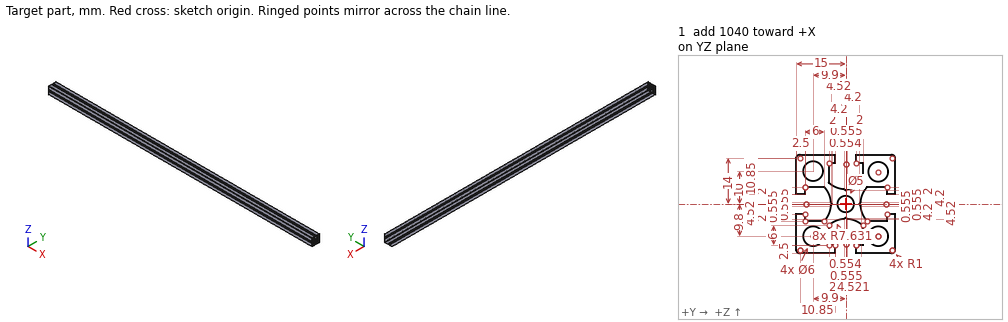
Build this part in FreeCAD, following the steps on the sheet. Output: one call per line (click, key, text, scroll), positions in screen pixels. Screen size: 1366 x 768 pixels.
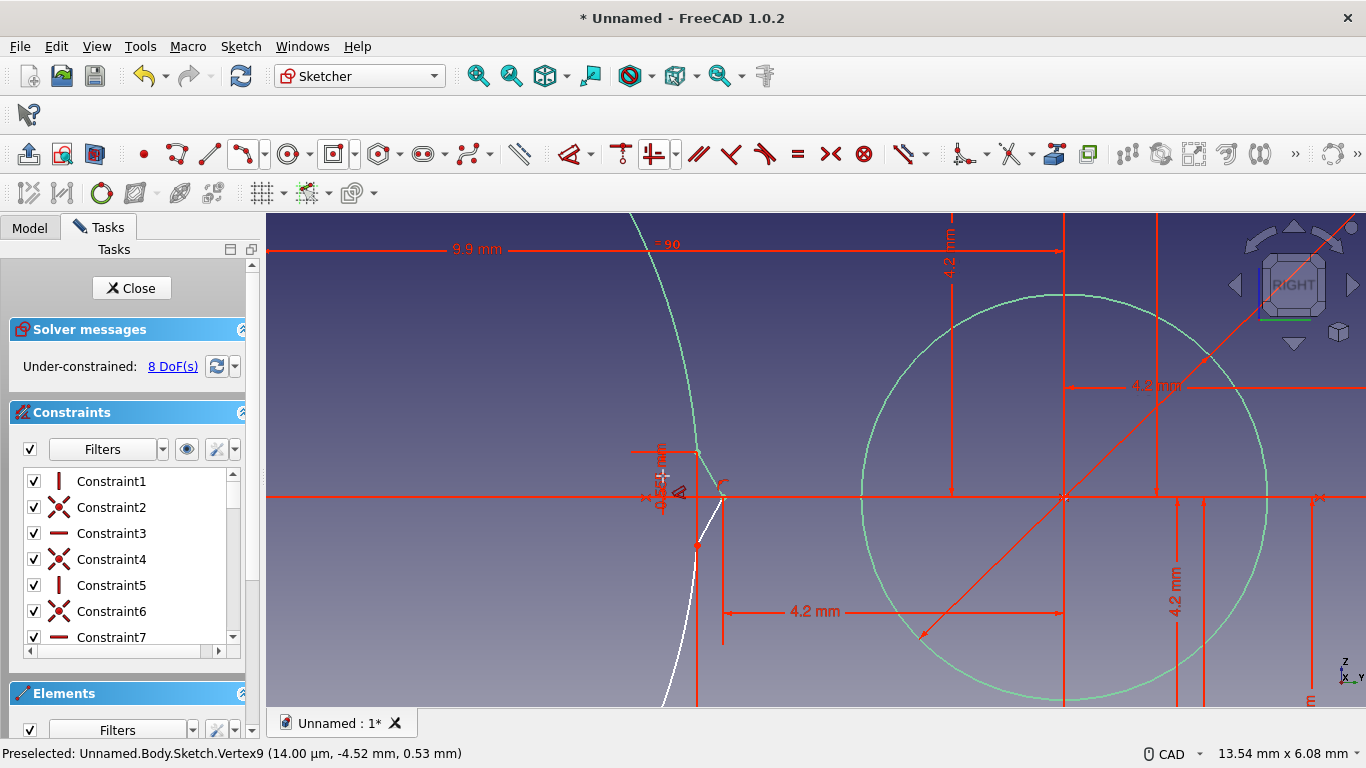
click(697, 545)
click(663, 521)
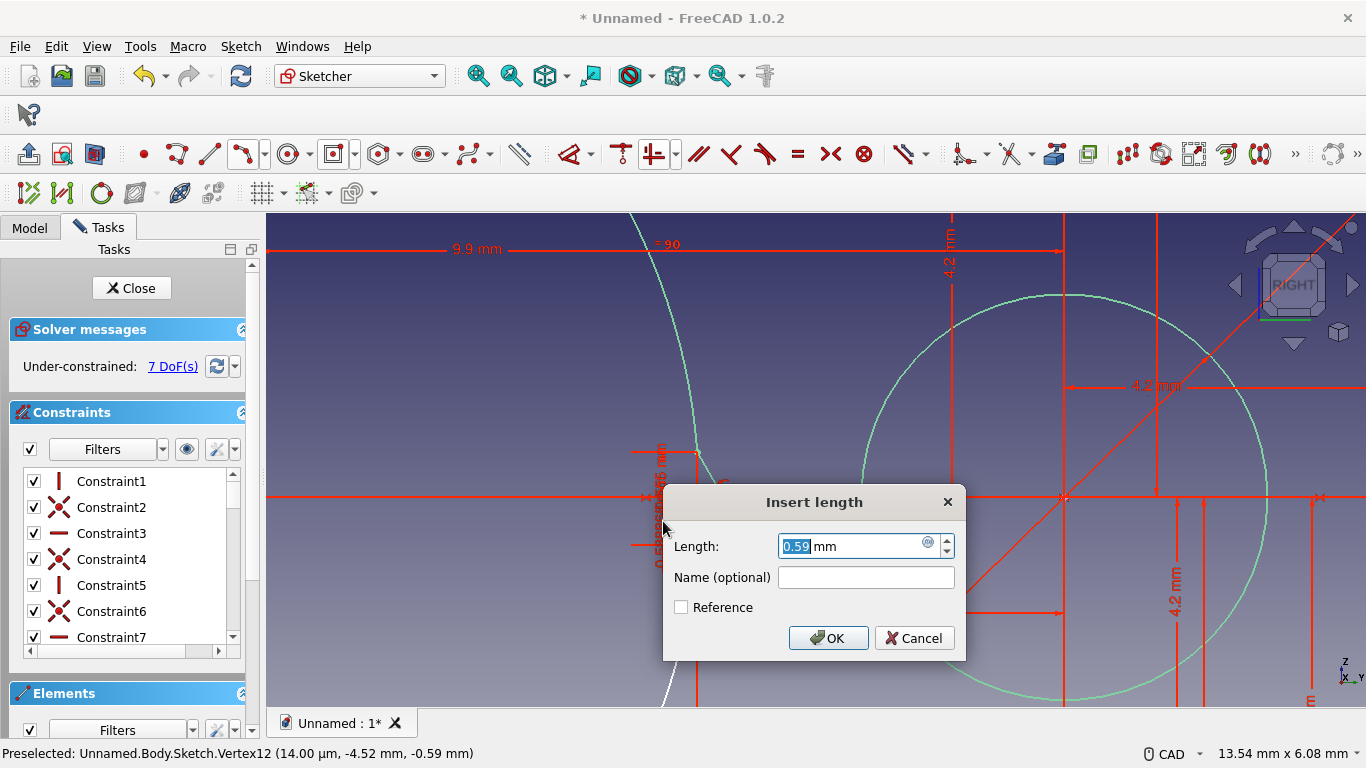
text(0.555)
key(Return)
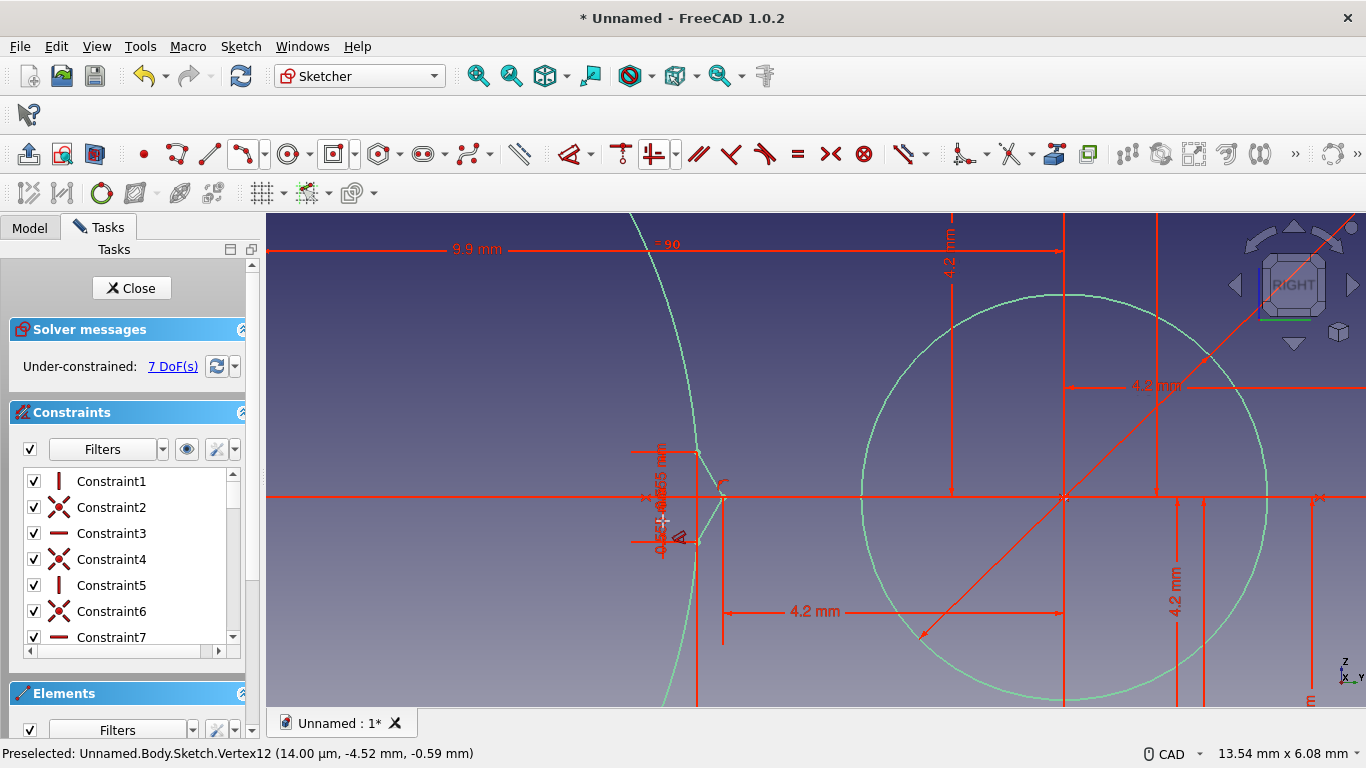
scroll(698, 454, down, 10)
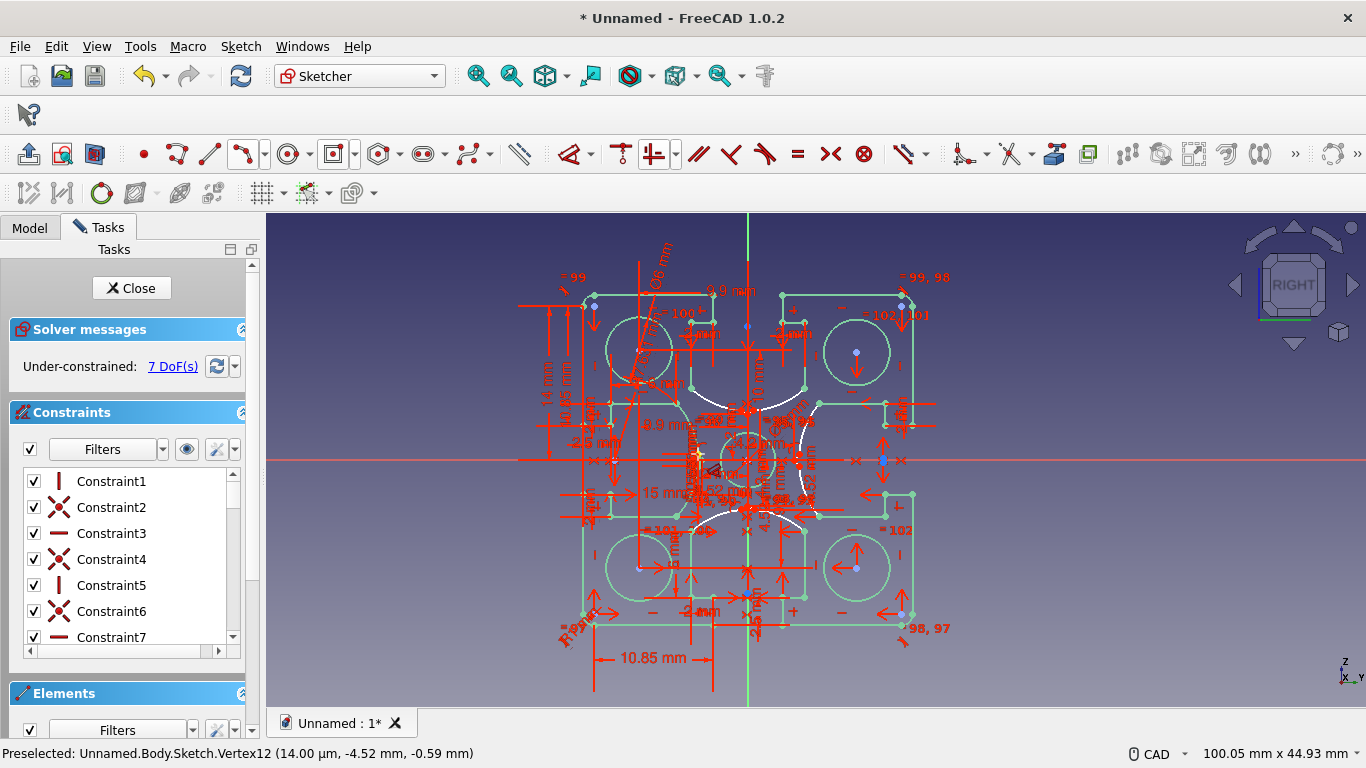
scroll(742, 510, up, 10)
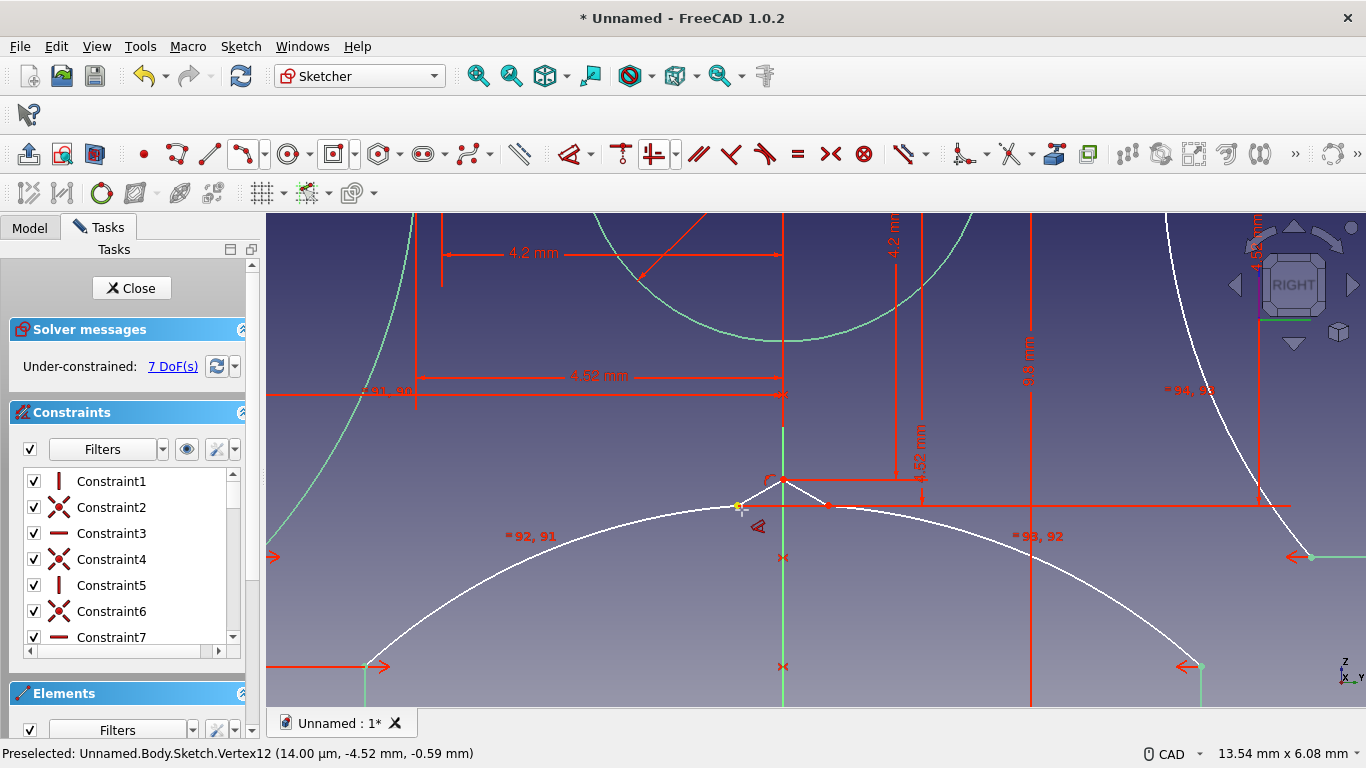
click(738, 506)
click(760, 540)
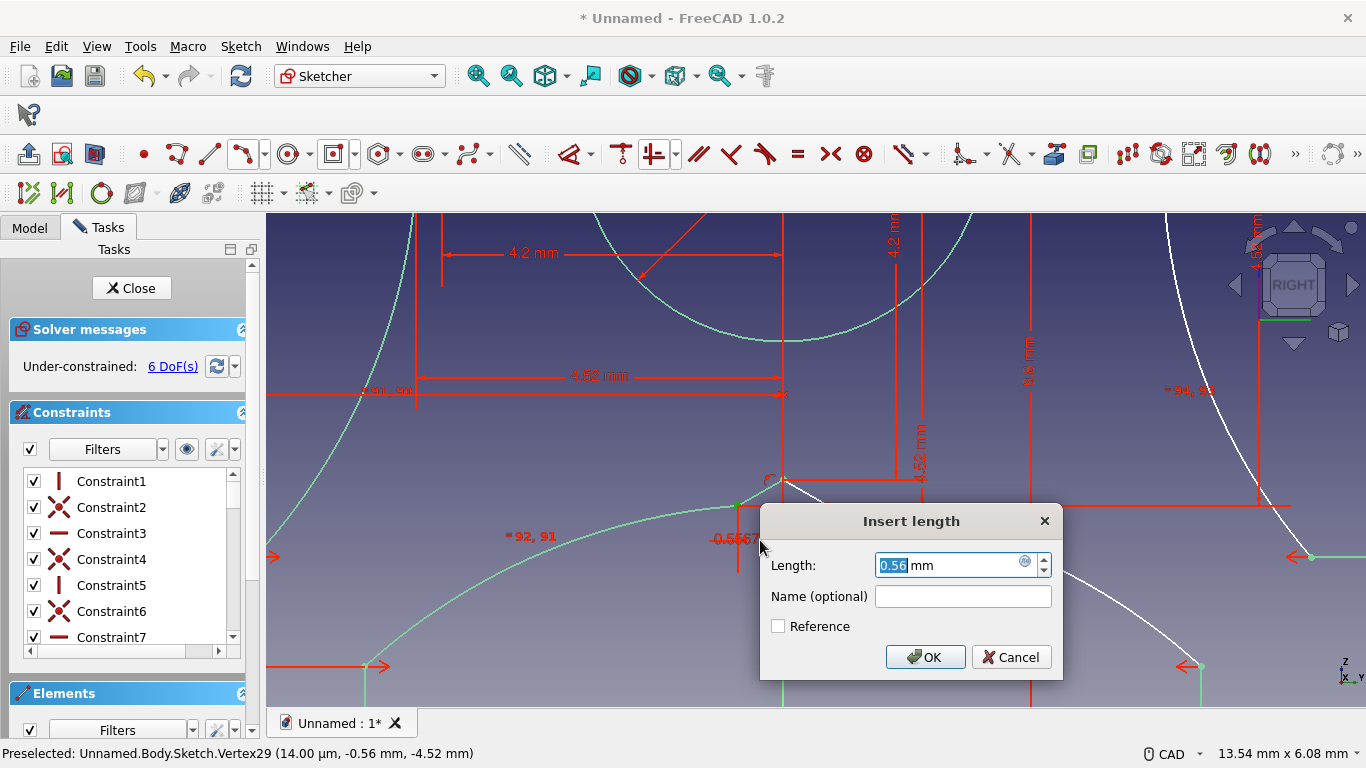
text(0.554)
key(Return)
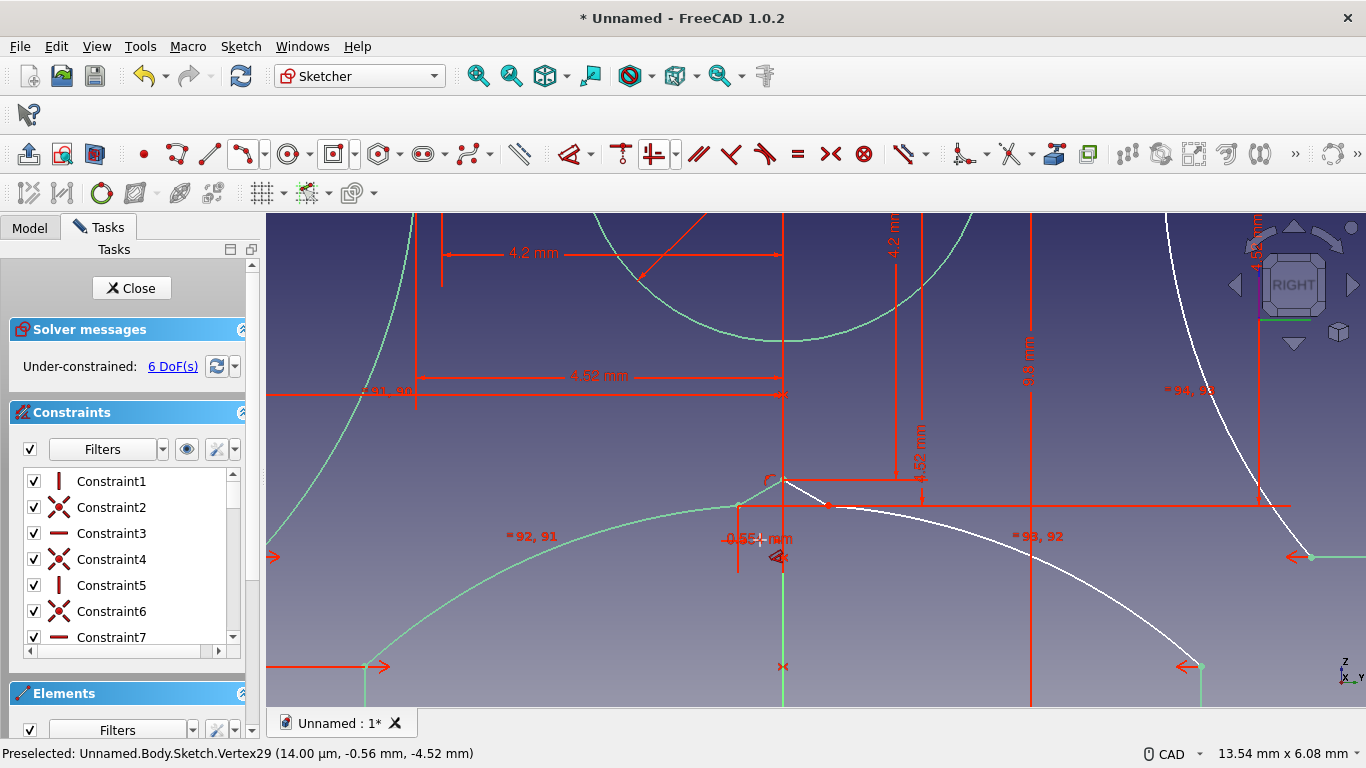
click(828, 506)
click(806, 564)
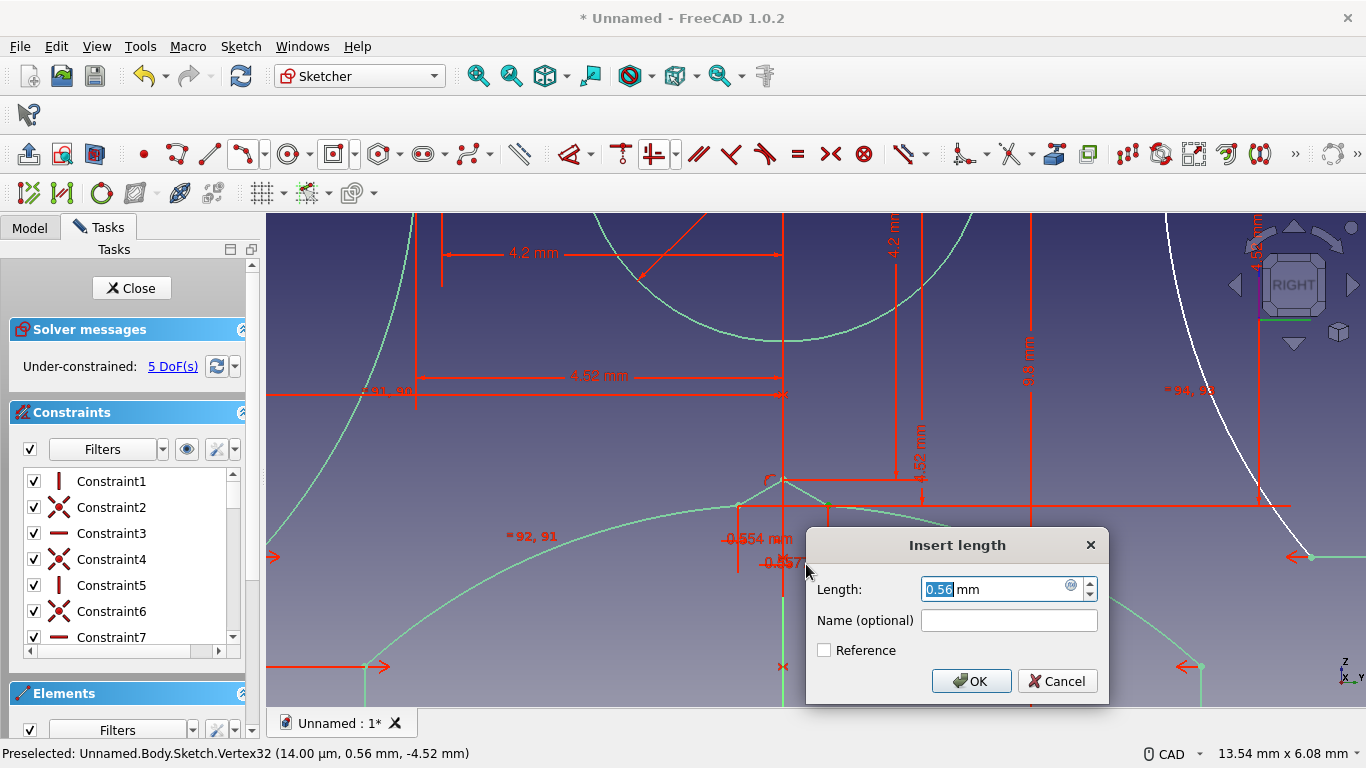
text(0.555)
key(Return)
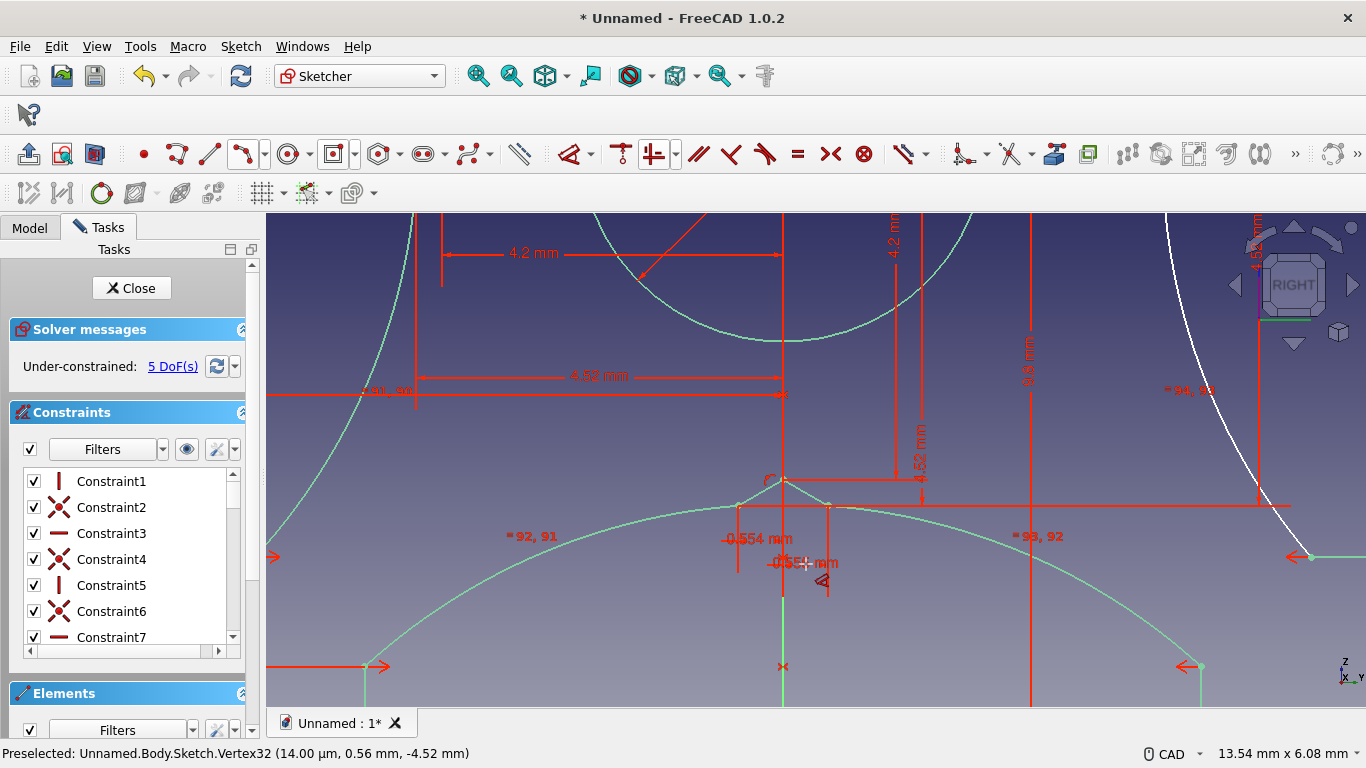
scroll(742, 510, down, 10)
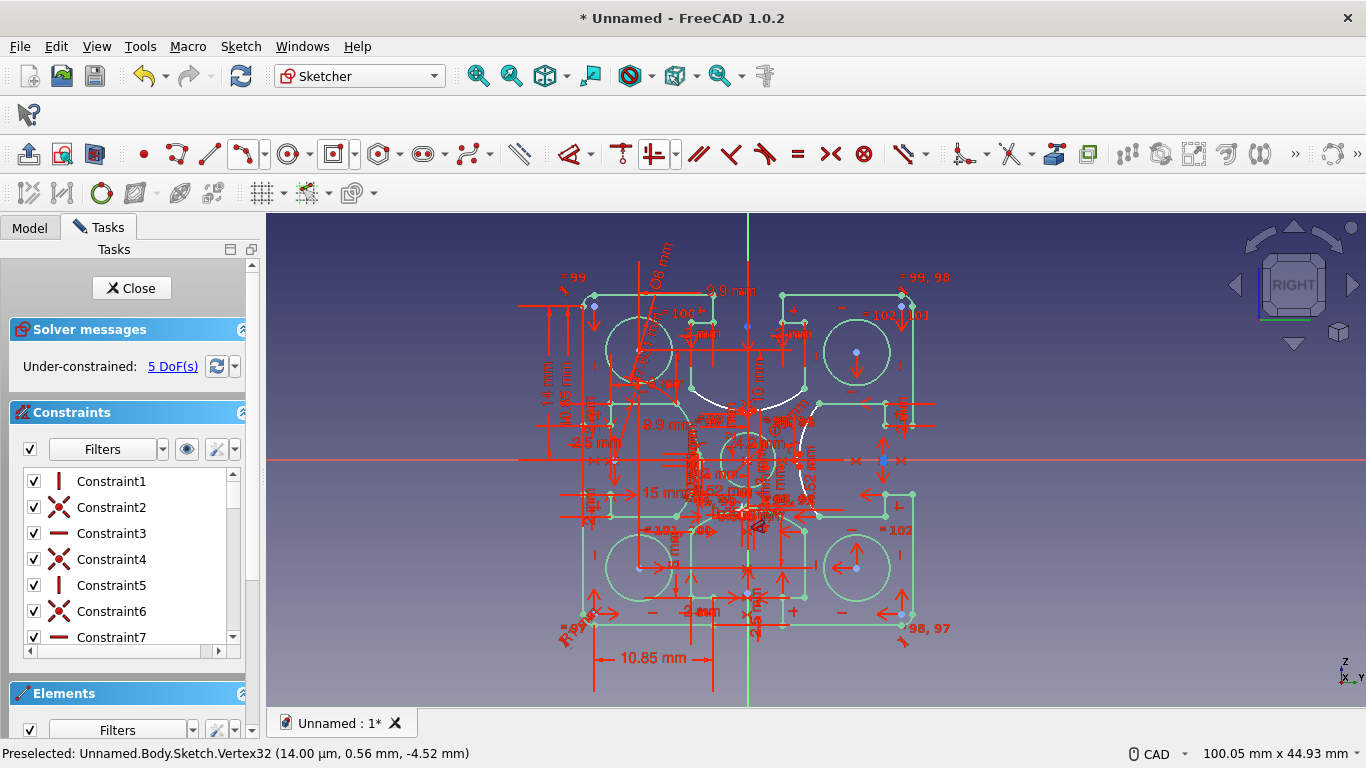
scroll(799, 467, up, 2)